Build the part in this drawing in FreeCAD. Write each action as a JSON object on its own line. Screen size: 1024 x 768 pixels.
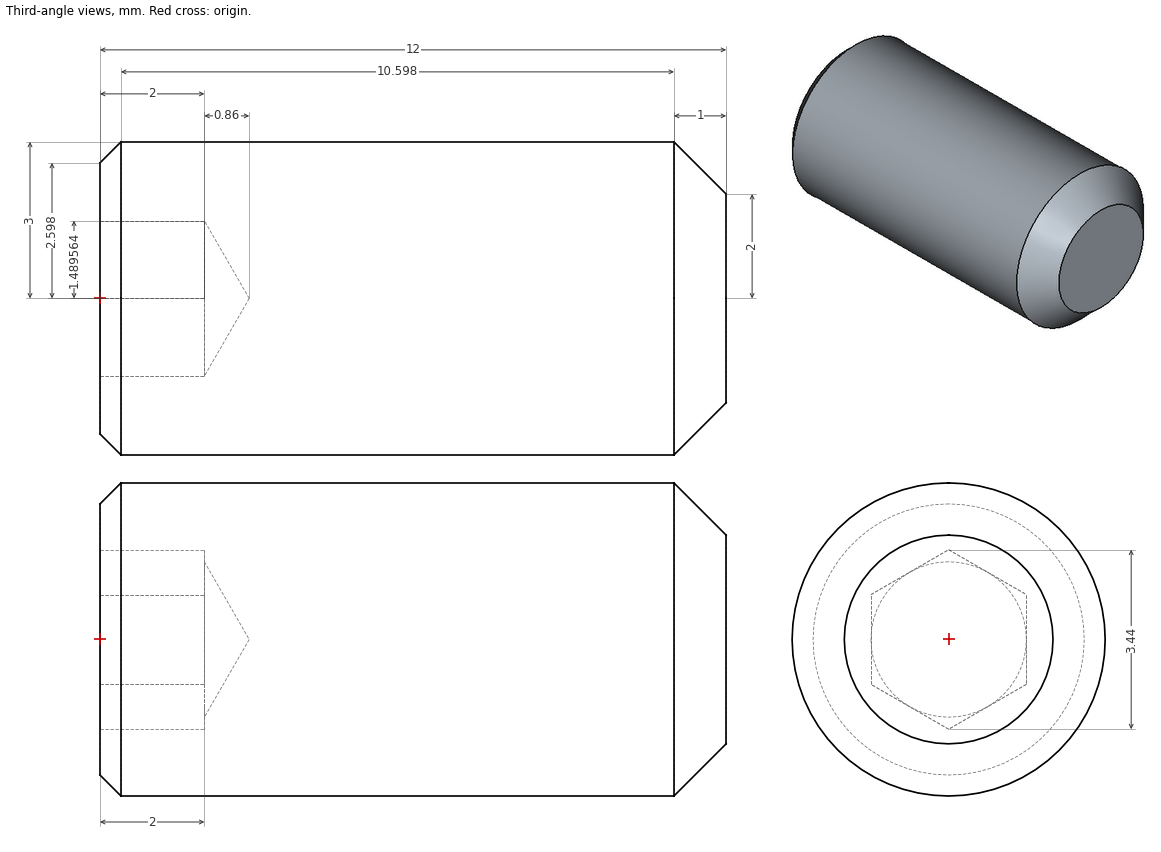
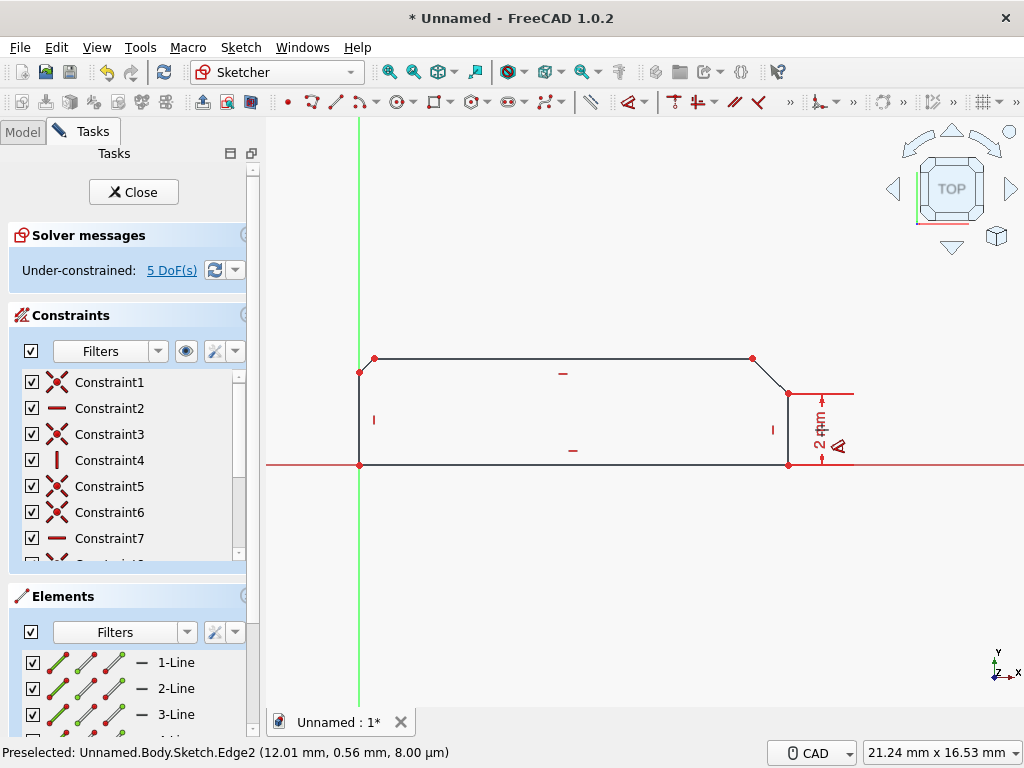
{"action": "left_click", "coordinate": [488, 465]}
{"action": "left_click", "coordinate": [574, 499]}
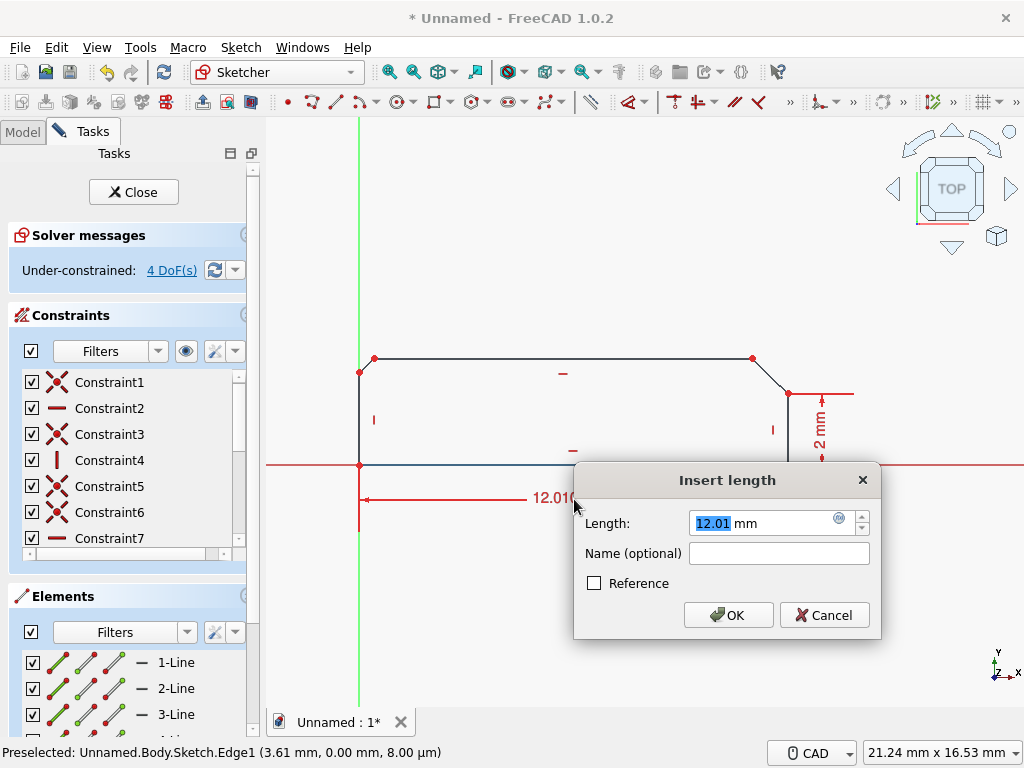
{"action": "type", "text": "12"}
{"action": "key", "text": "Return"}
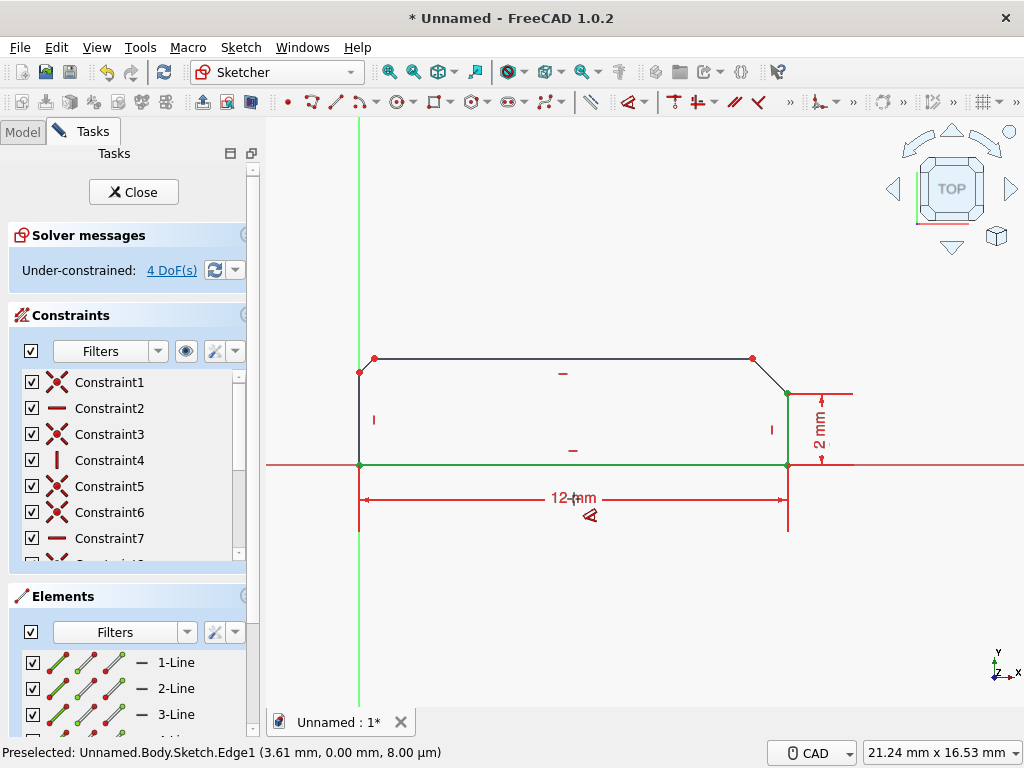
{"action": "left_click", "coordinate": [752, 359]}
{"action": "left_click", "coordinate": [325, 412]}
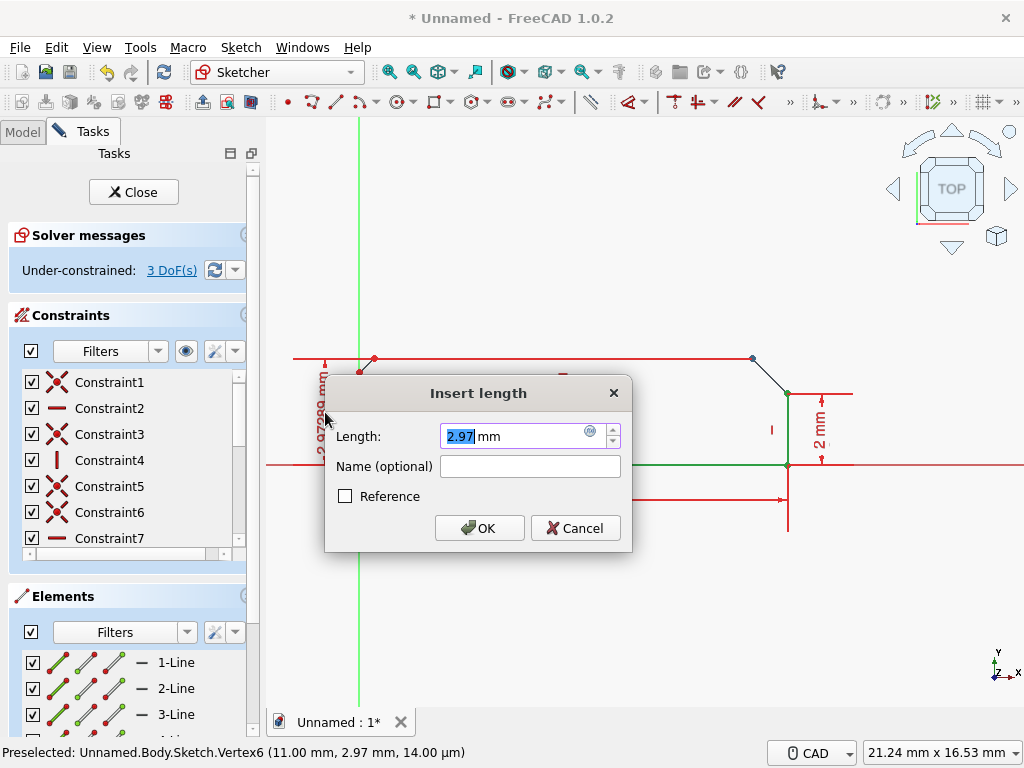
{"action": "type", "text": "3"}
{"action": "key", "text": "Return"}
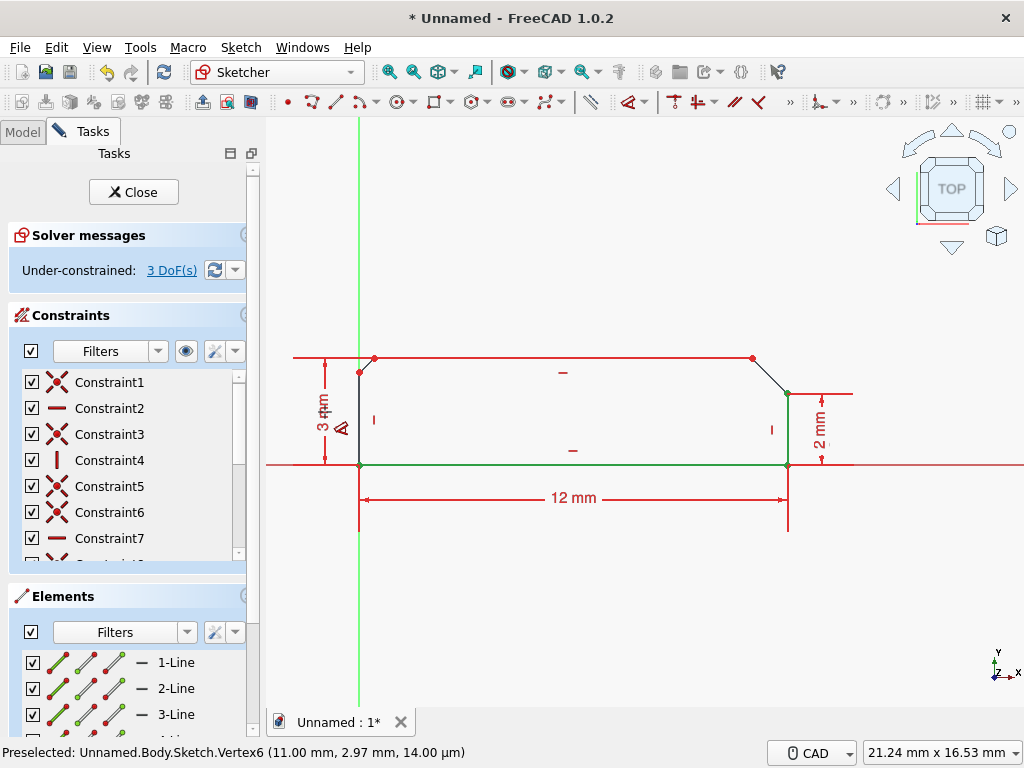
{"action": "left_click", "coordinate": [777, 383]}
{"action": "left_click", "coordinate": [770, 324]}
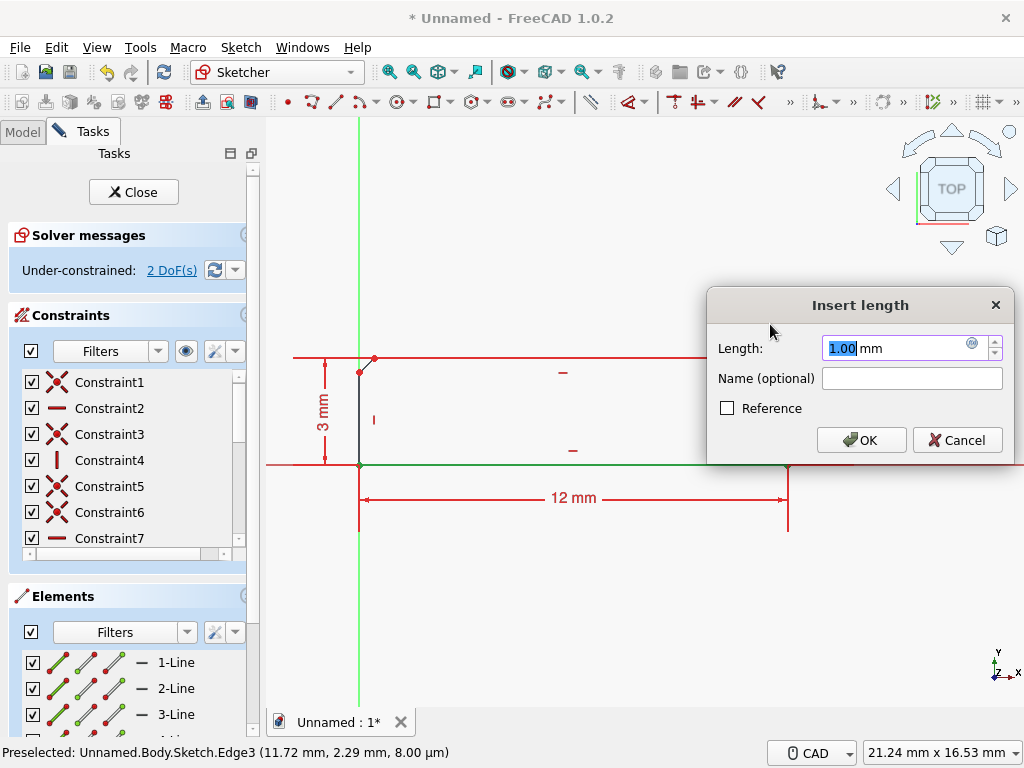
{"action": "type", "text": "1"}
{"action": "key", "text": "Return"}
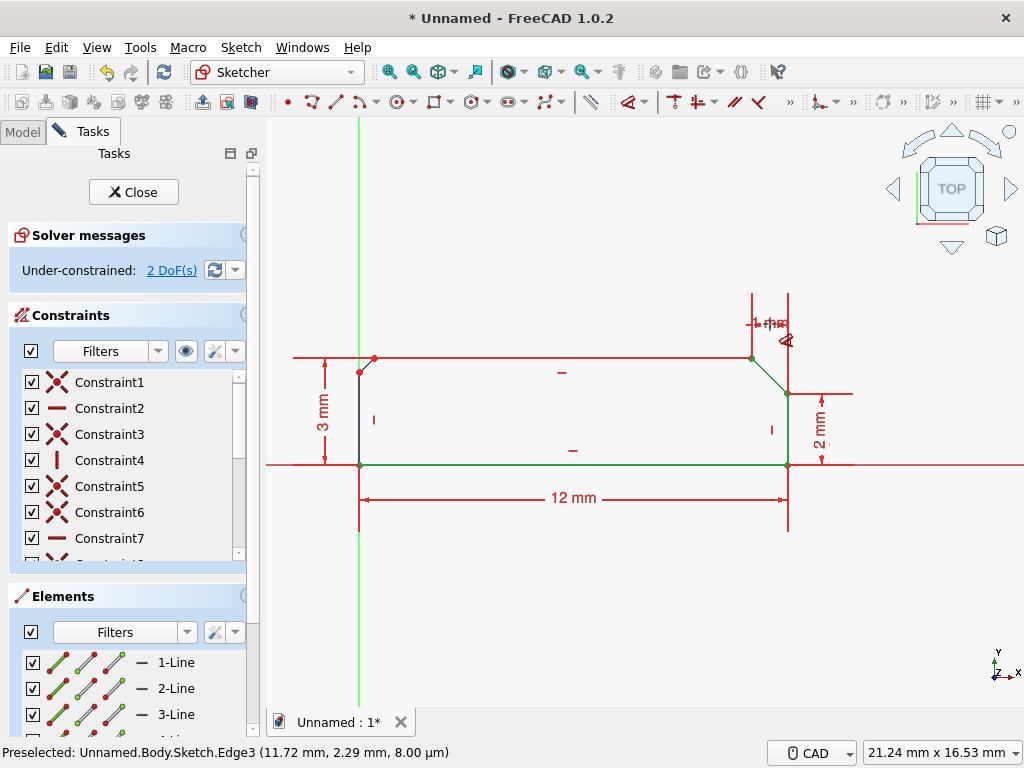
{"action": "left_click", "coordinate": [359, 401]}
{"action": "left_click", "coordinate": [325, 440]}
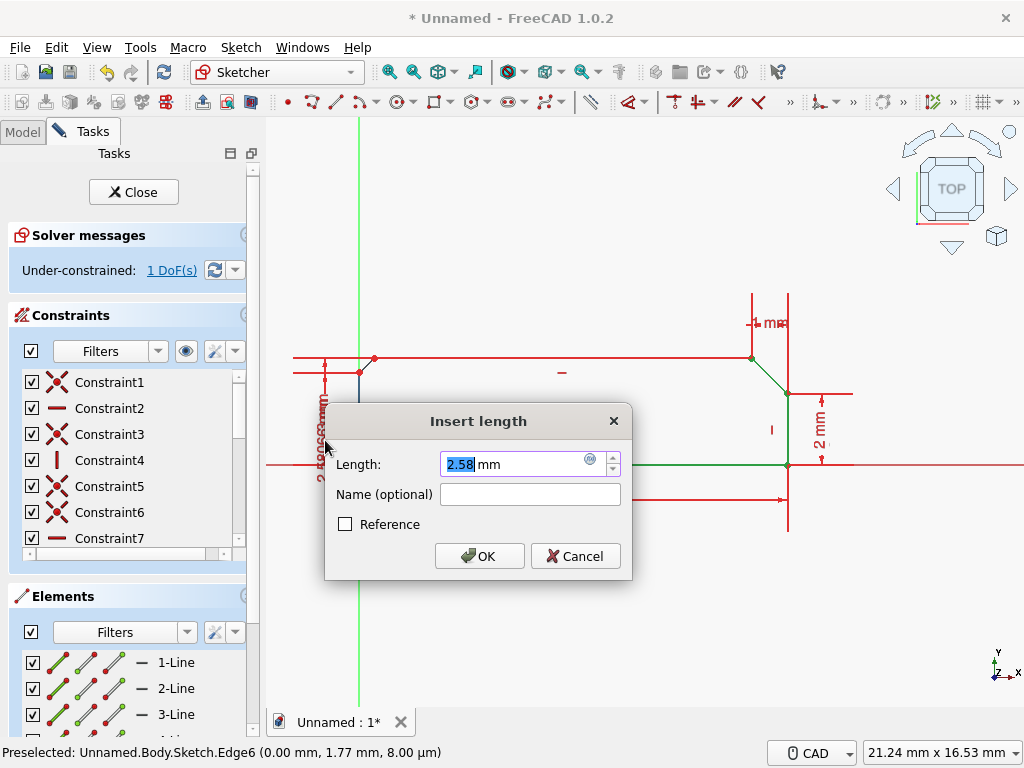
{"action": "type", "text": "2.598"}
{"action": "key", "text": "Return"}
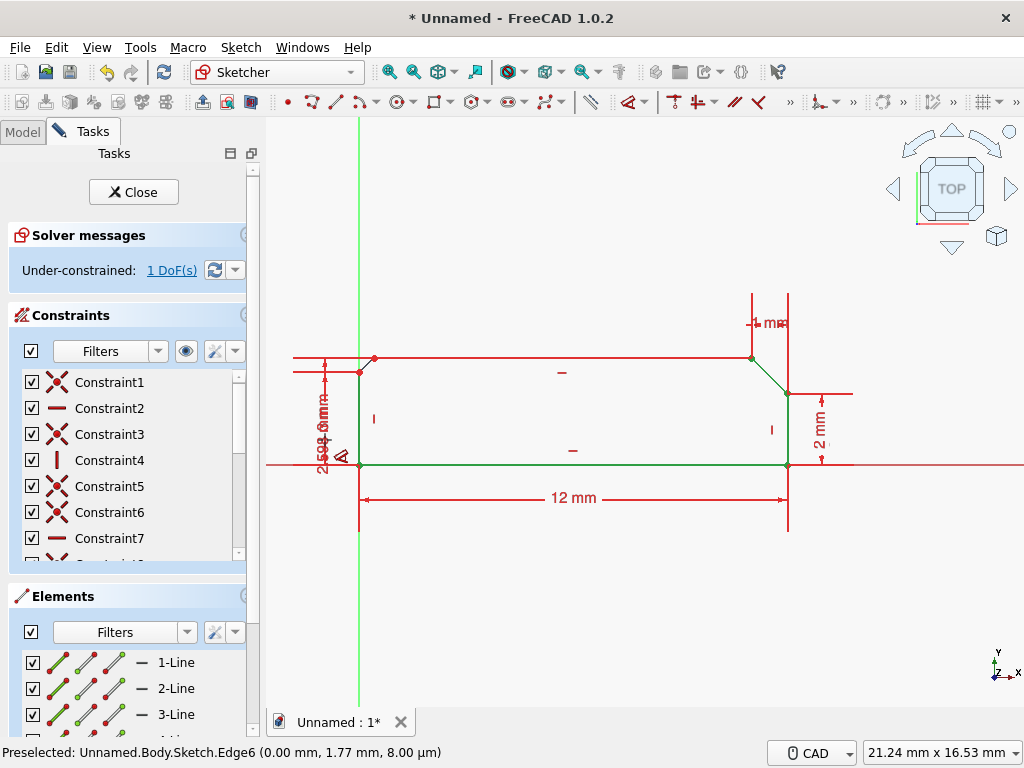
{"action": "left_click", "coordinate": [639, 358]}
{"action": "left_click", "coordinate": [563, 324]}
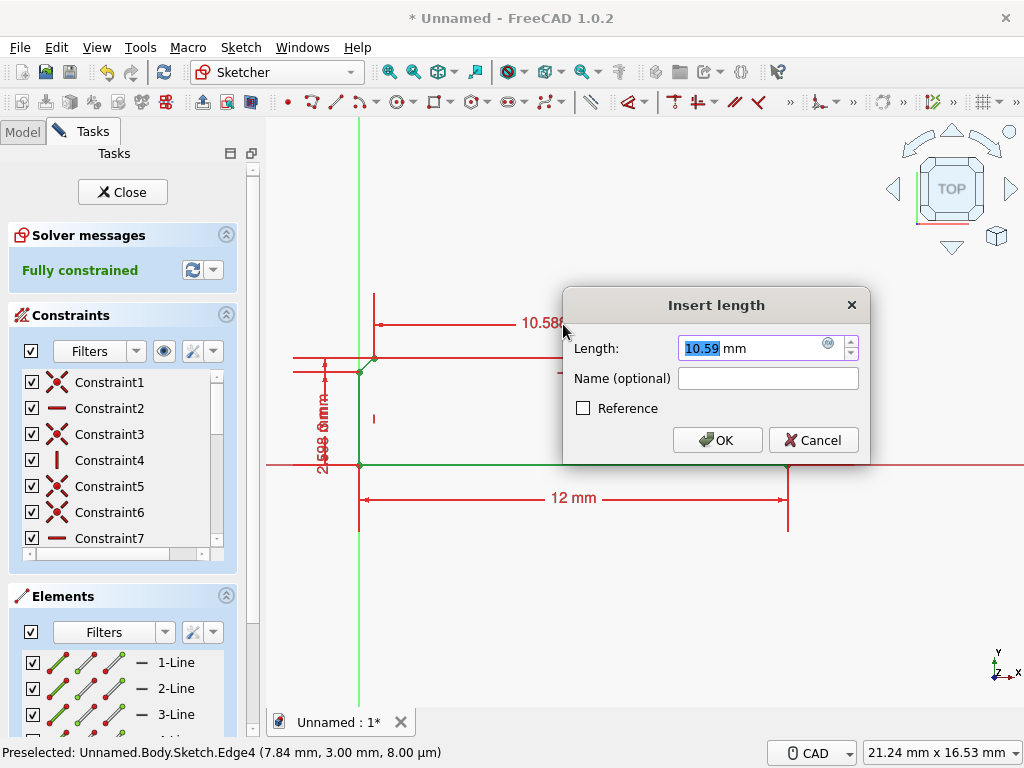
{"action": "type", "text": "10.598"}
{"action": "key", "text": "Return"}
{"action": "key", "text": "Escape"}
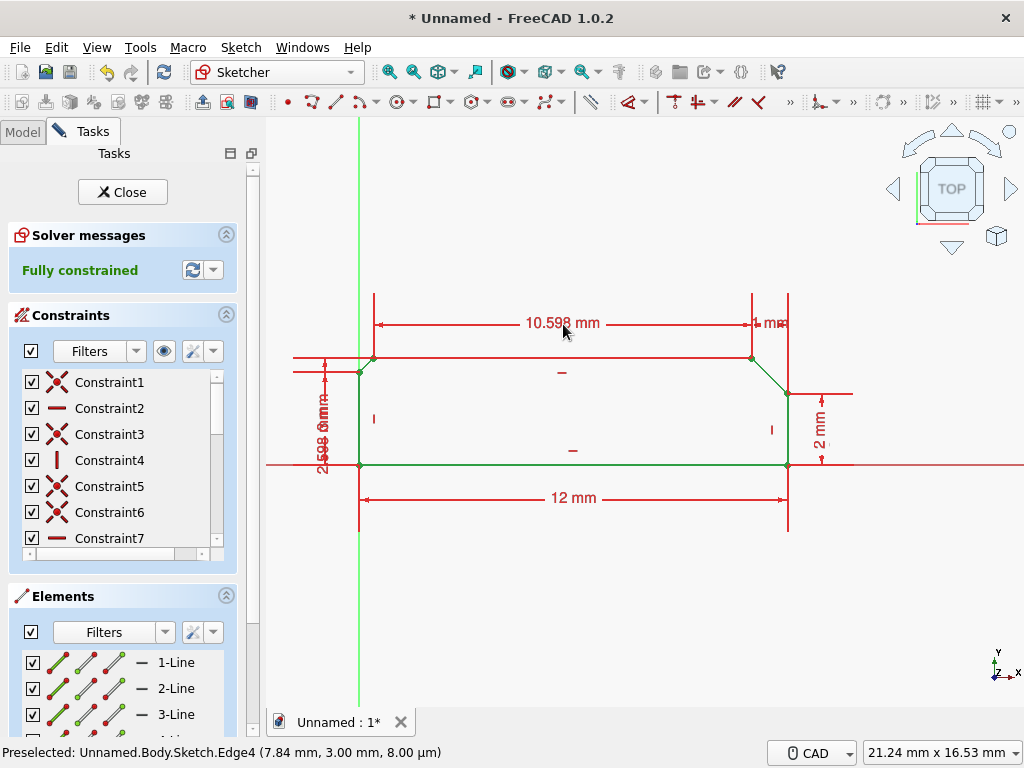
{"action": "left_click", "coordinate": [123, 192]}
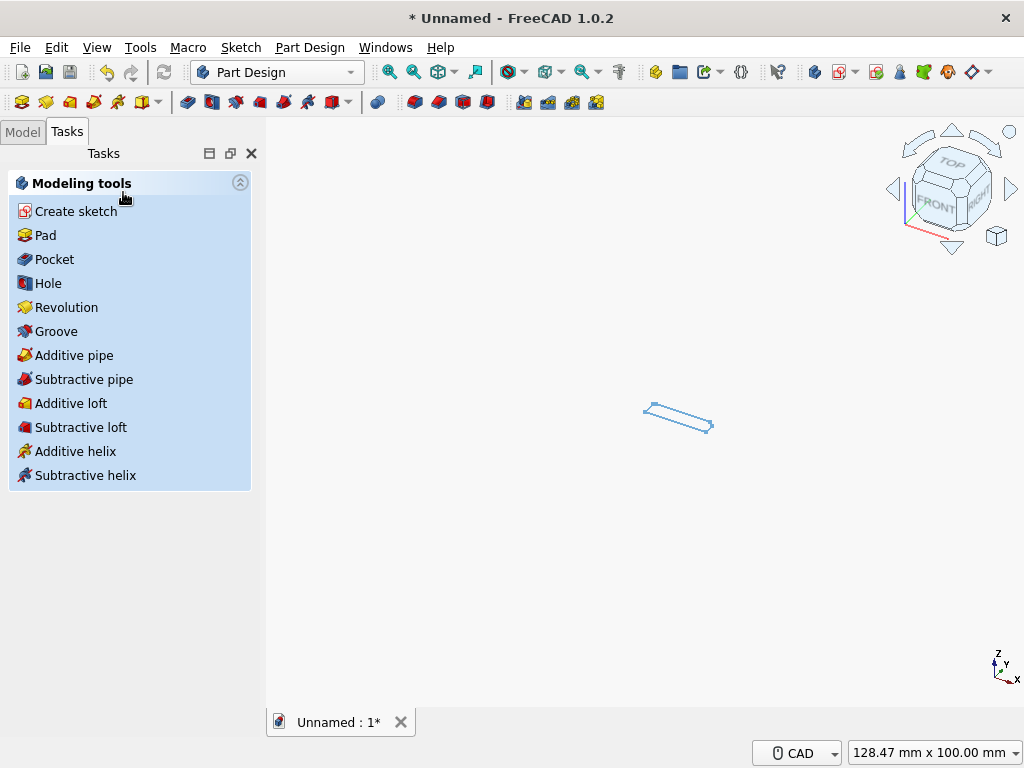
{"action": "left_click", "coordinate": [46, 102]}